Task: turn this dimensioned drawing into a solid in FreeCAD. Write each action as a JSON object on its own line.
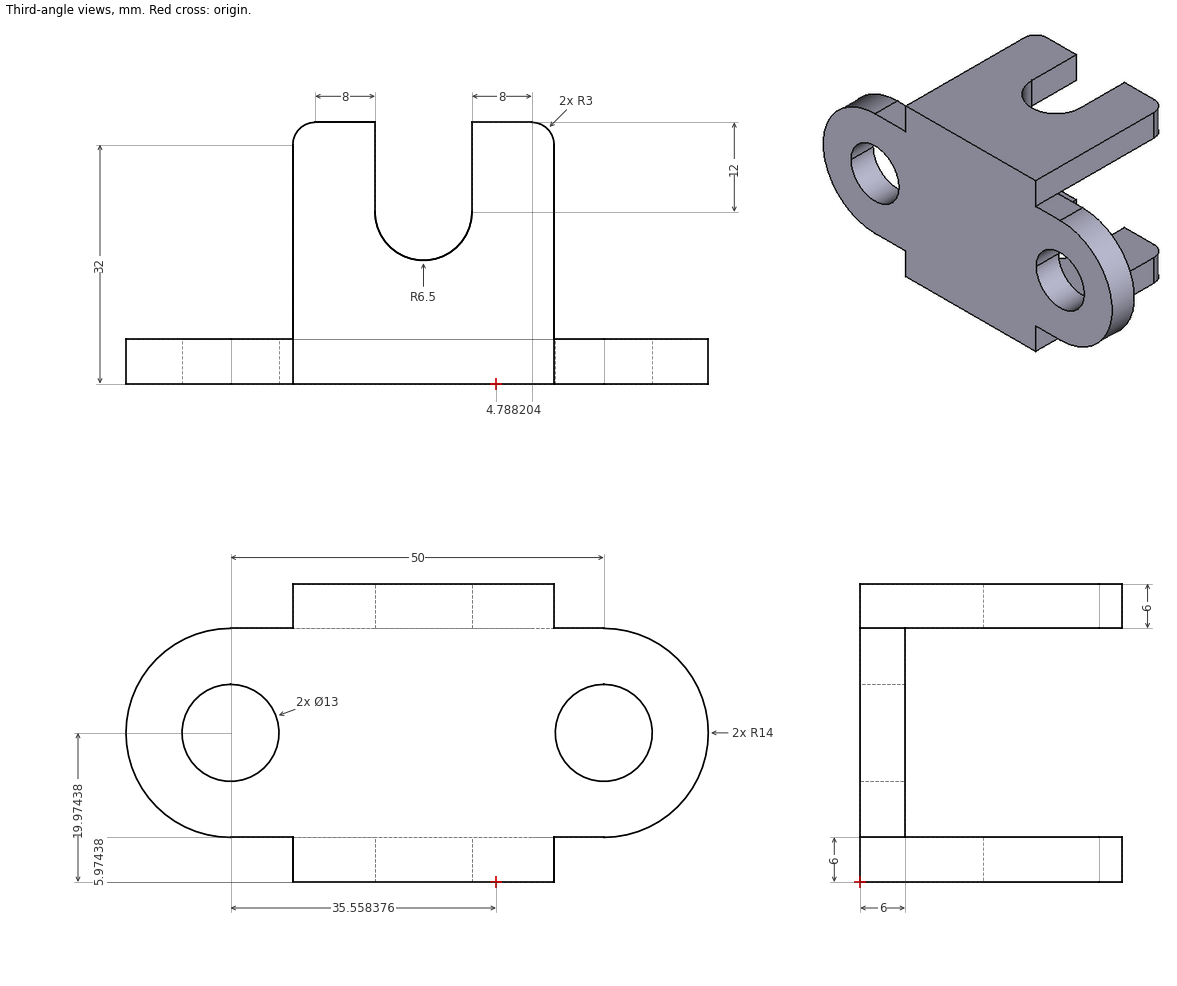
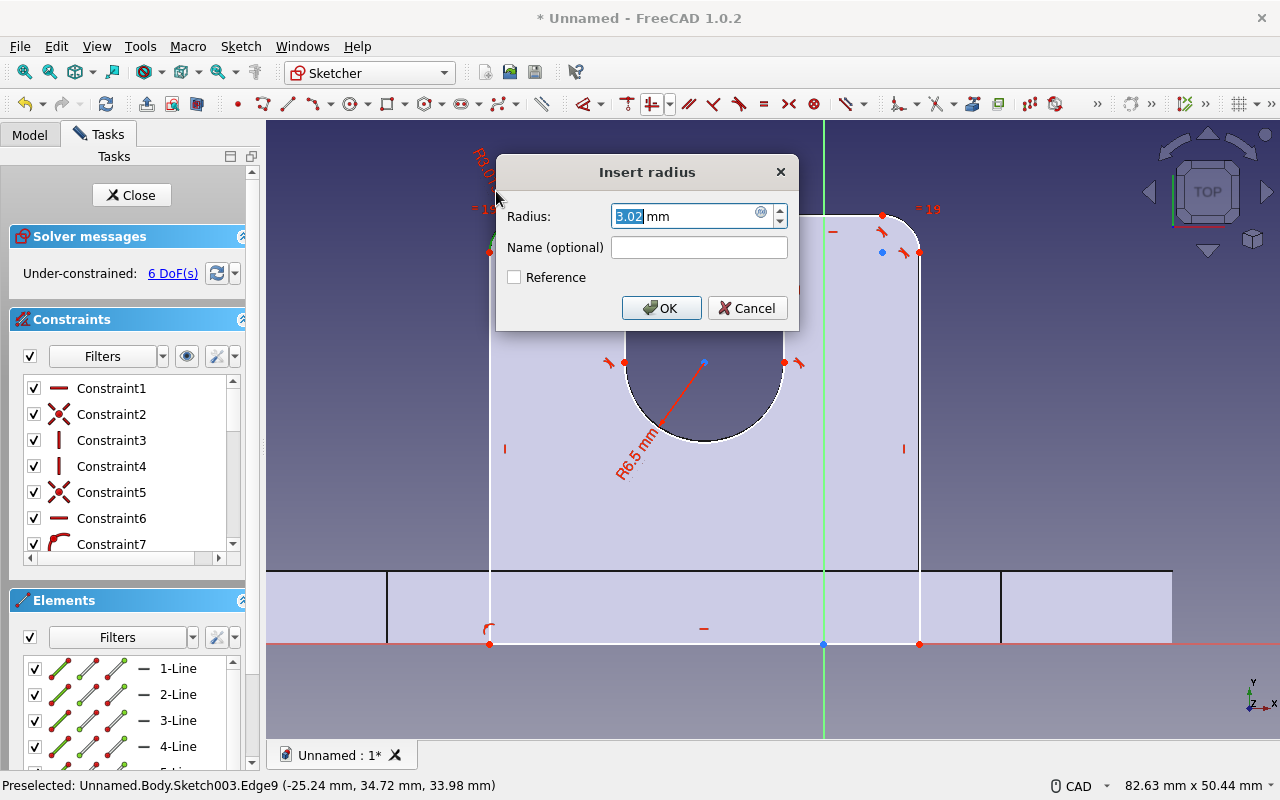
{"action": "type", "text": "3"}
{"action": "key", "text": "Return"}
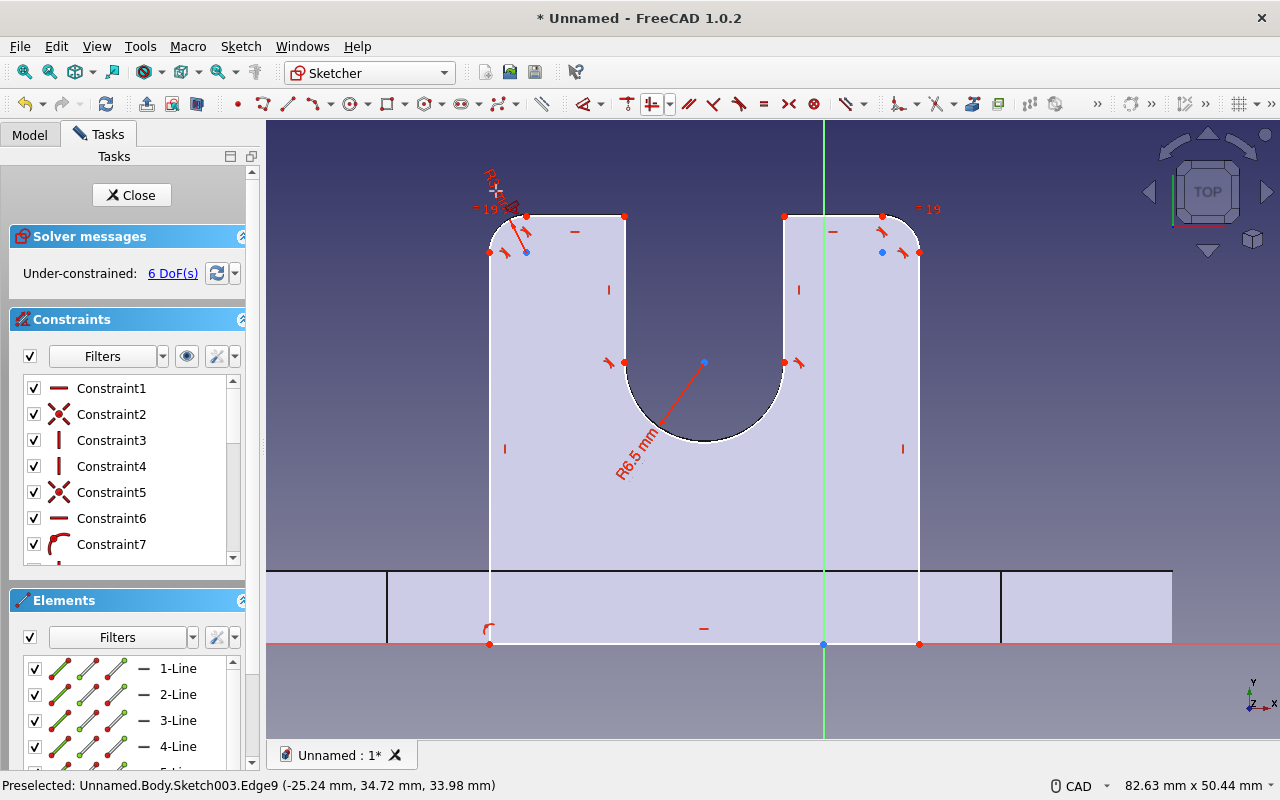
{"action": "left_click", "coordinate": [853, 216]}
{"action": "left_click", "coordinate": [811, 182]}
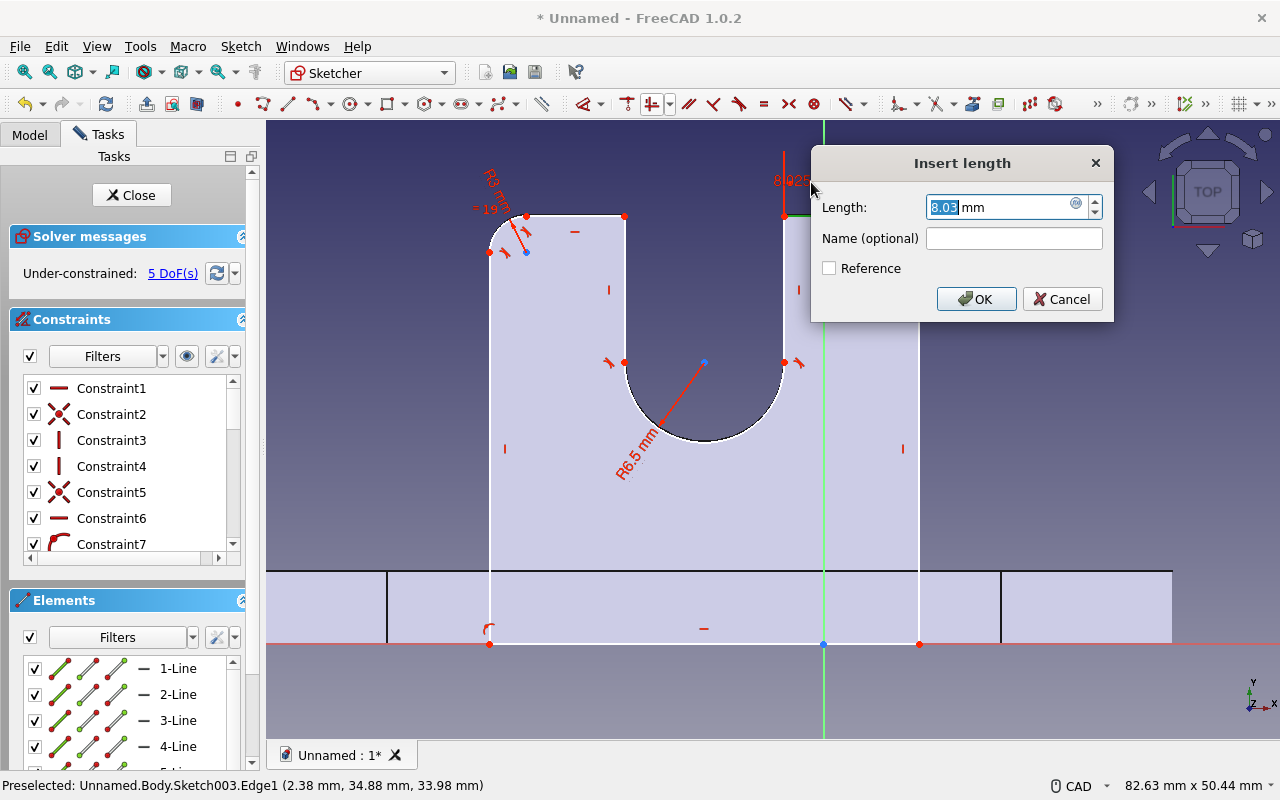
{"action": "type", "text": "8"}
{"action": "key", "text": "Return"}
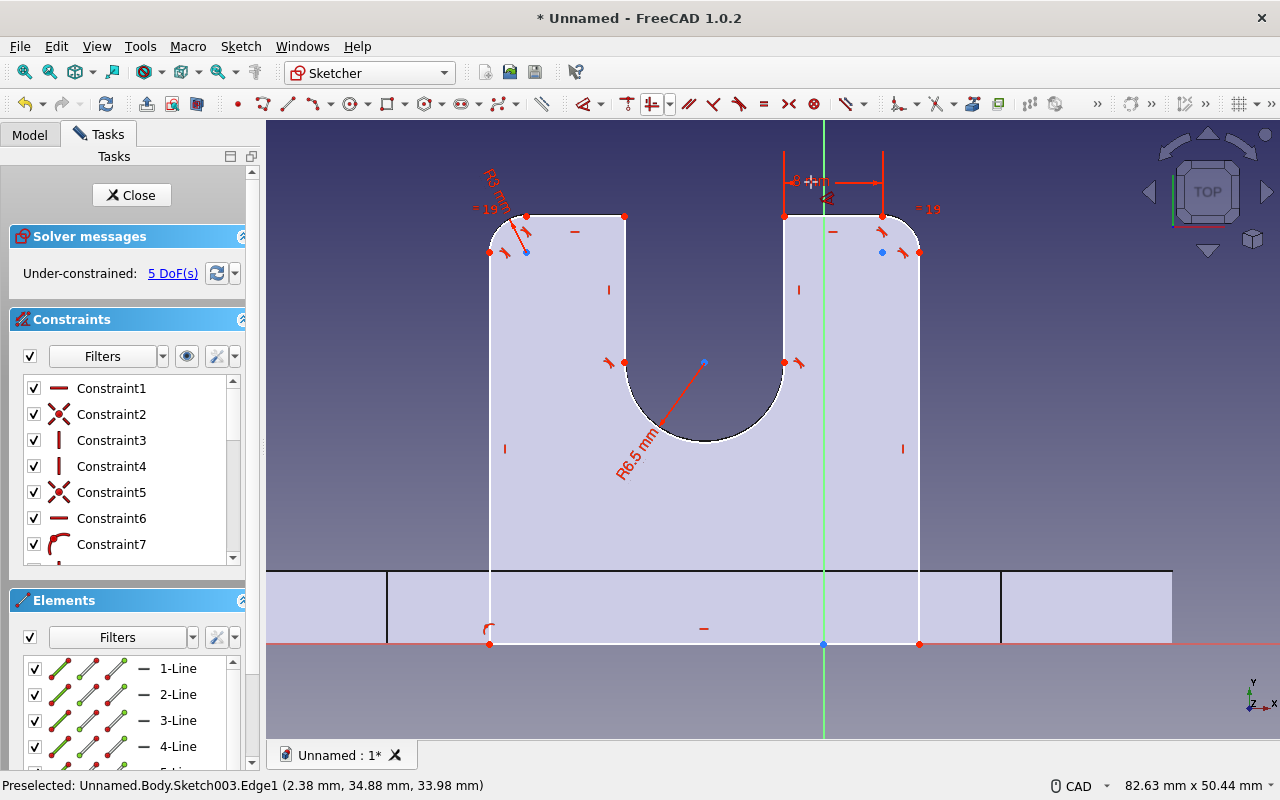
{"action": "left_click", "coordinate": [595, 216]}
{"action": "left_click", "coordinate": [576, 182]}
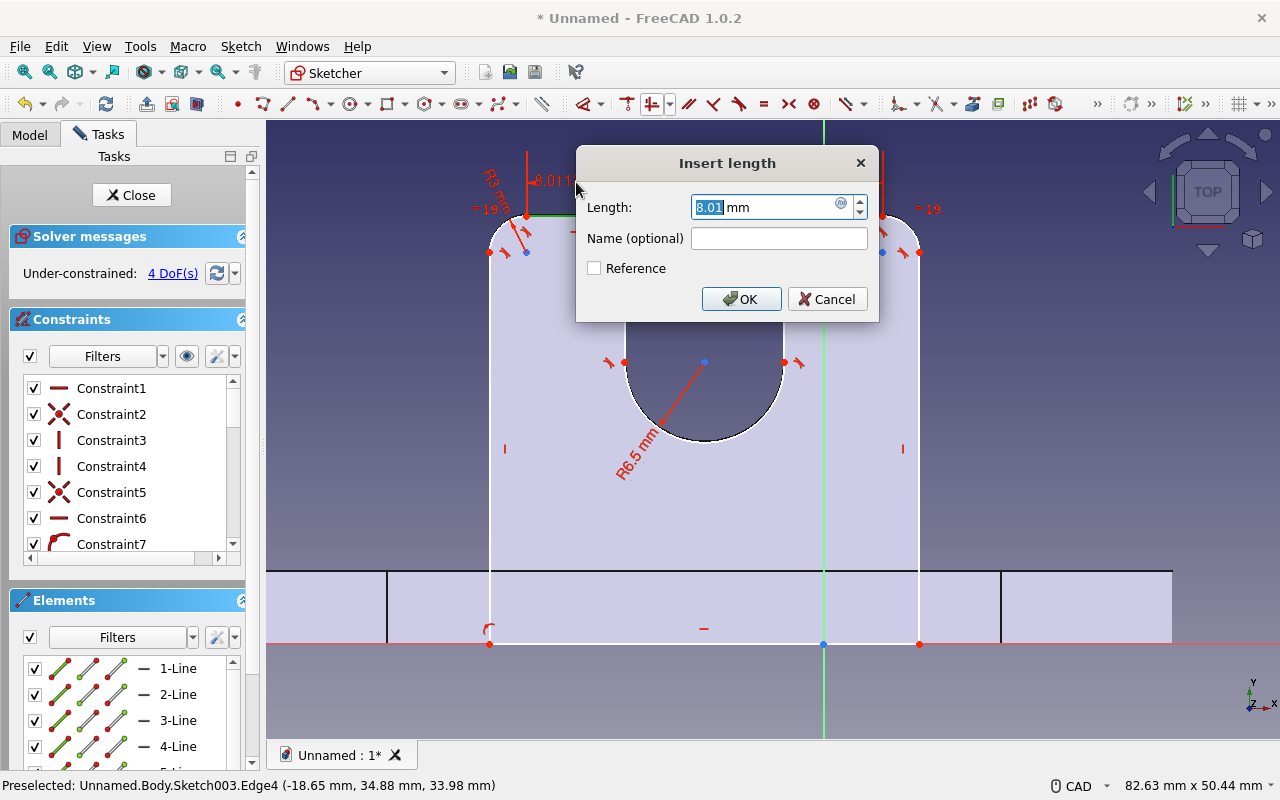
{"action": "type", "text": "8"}
{"action": "key", "text": "Return"}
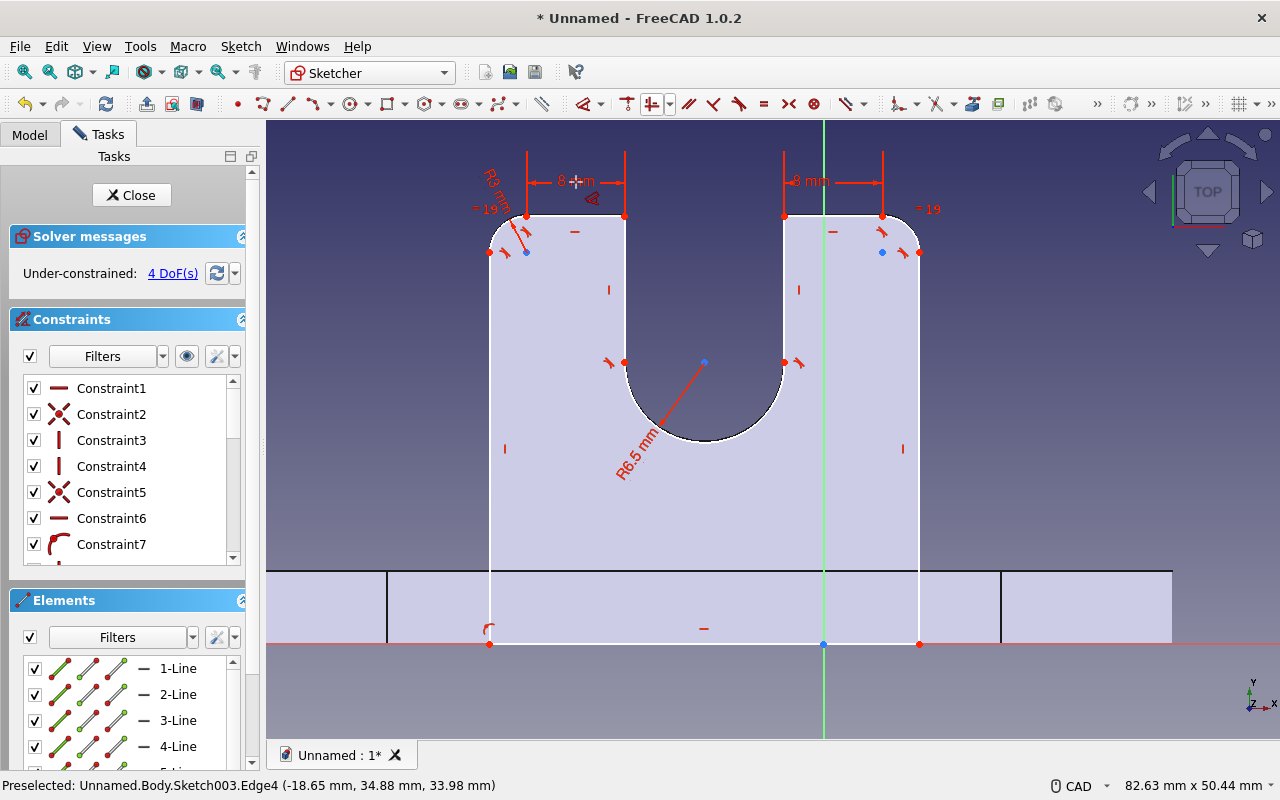
{"action": "left_click", "coordinate": [784, 260]}
{"action": "left_click", "coordinate": [750, 290]}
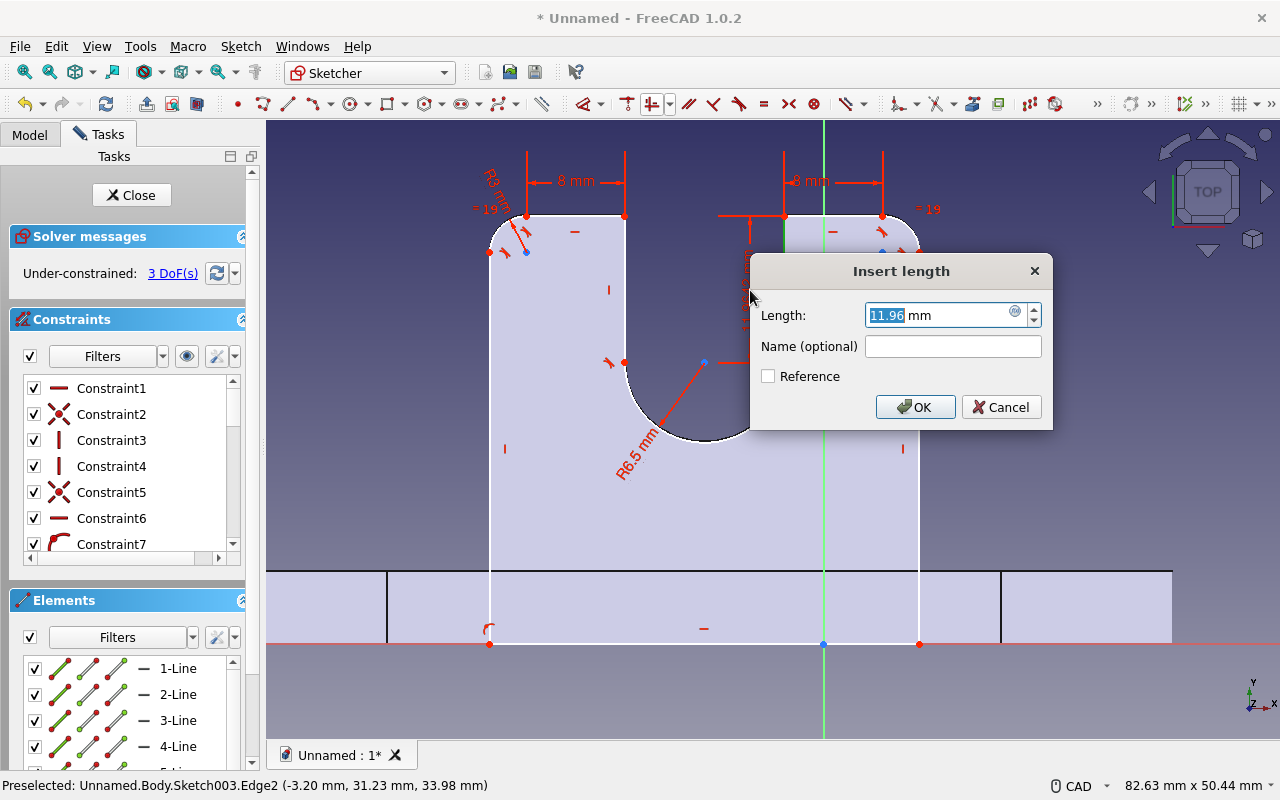
{"action": "type", "text": "12"}
{"action": "key", "text": "Return"}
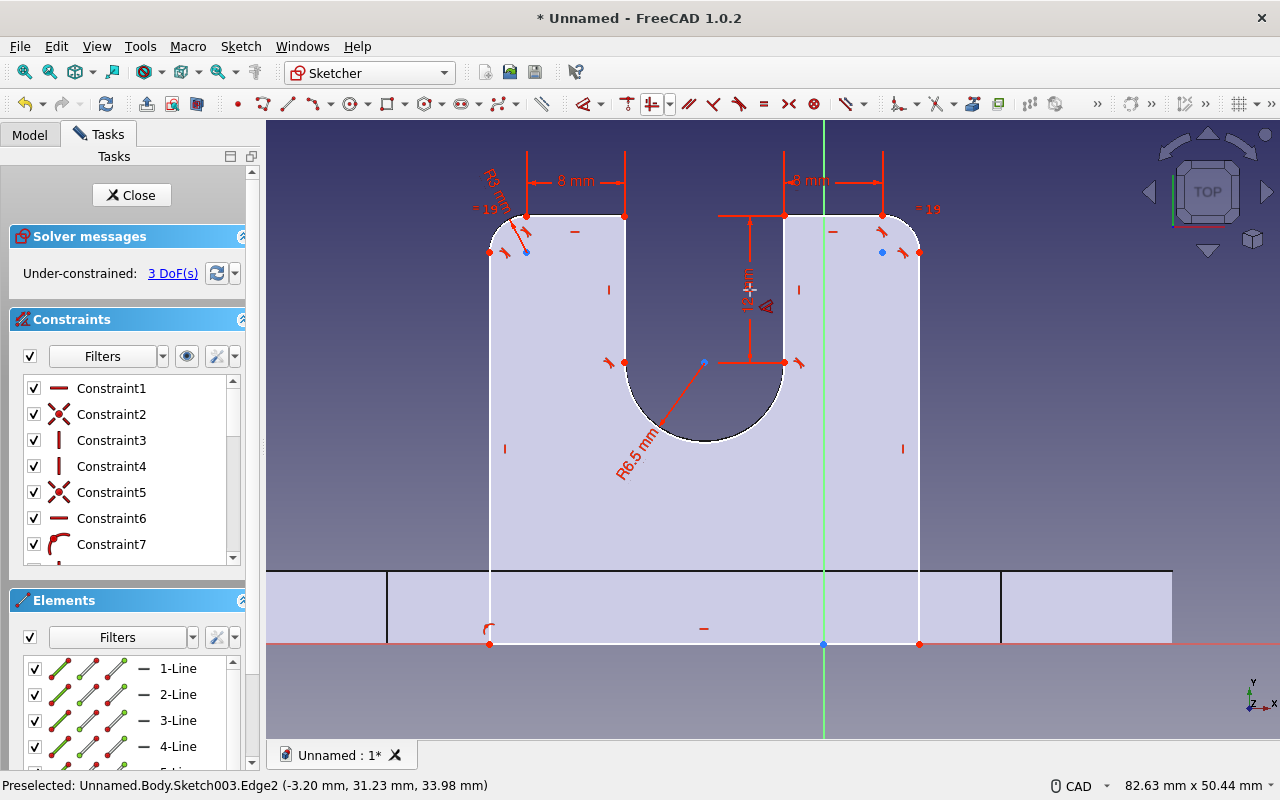
{"action": "left_click", "coordinate": [625, 319]}
{"action": "left_click", "coordinate": [591, 290]}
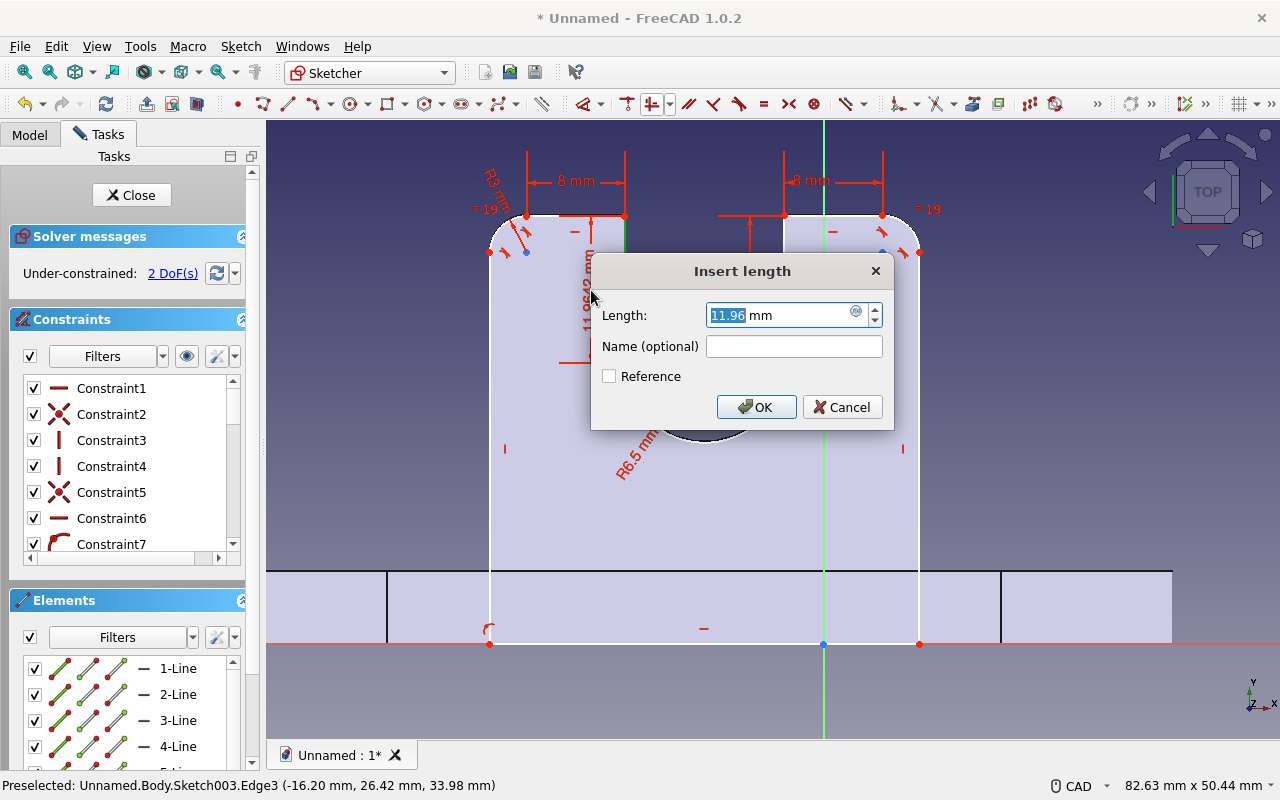
{"action": "type", "text": "12"}
{"action": "key", "text": "Return"}